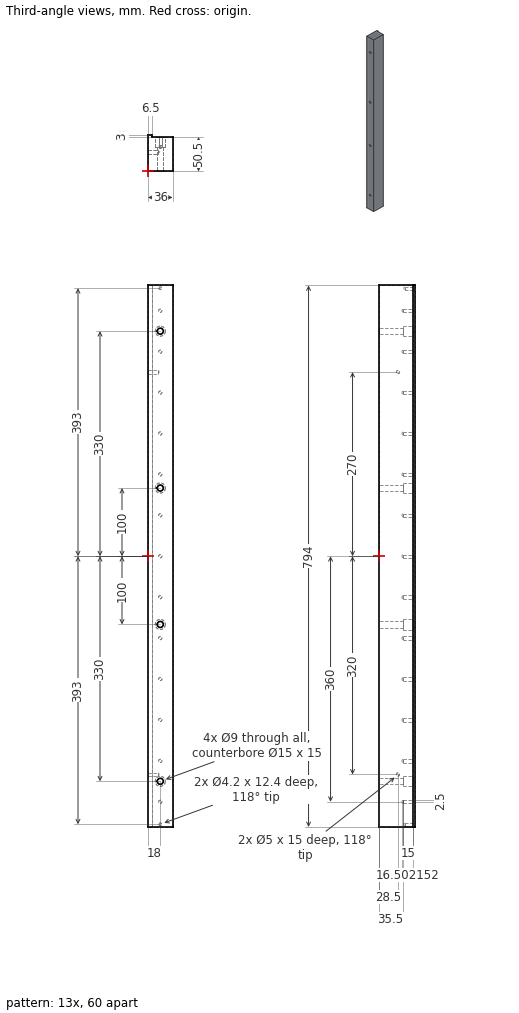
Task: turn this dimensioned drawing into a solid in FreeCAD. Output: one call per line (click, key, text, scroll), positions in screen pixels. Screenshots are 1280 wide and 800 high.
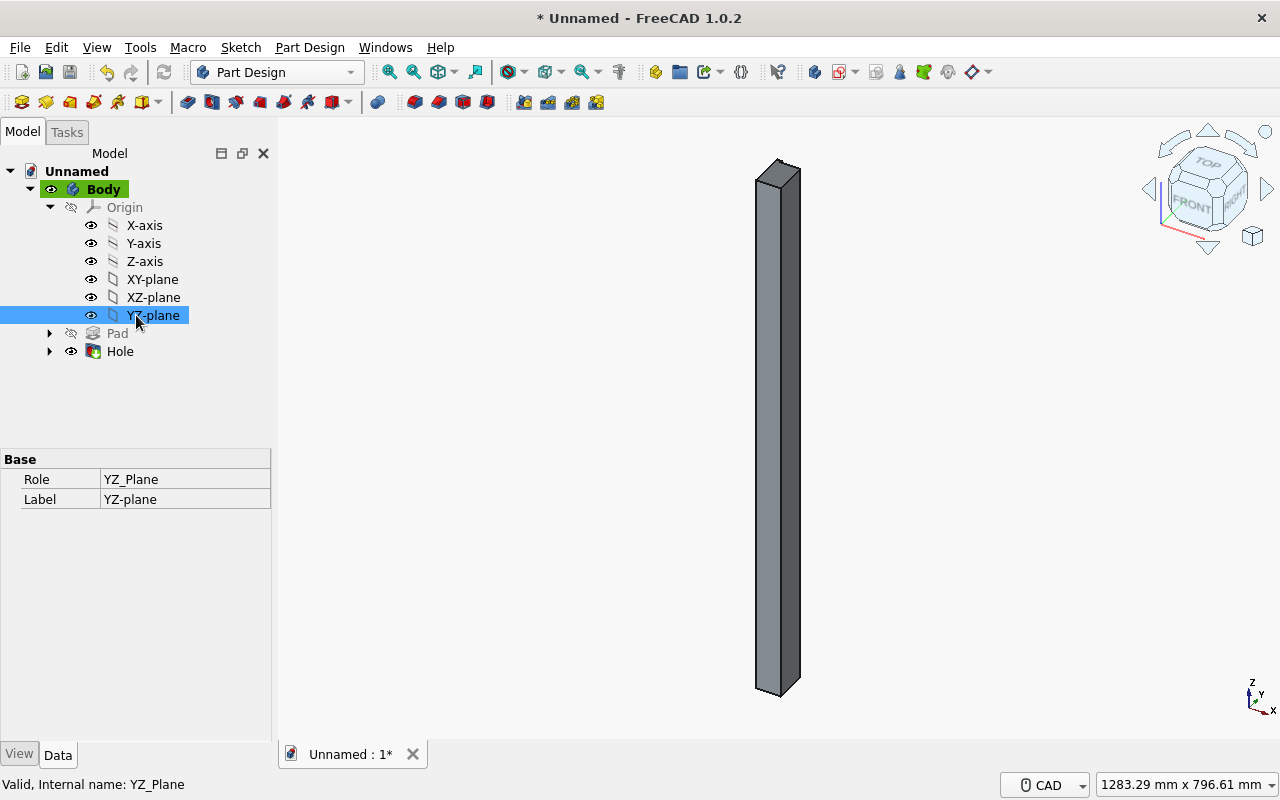
click(972, 72)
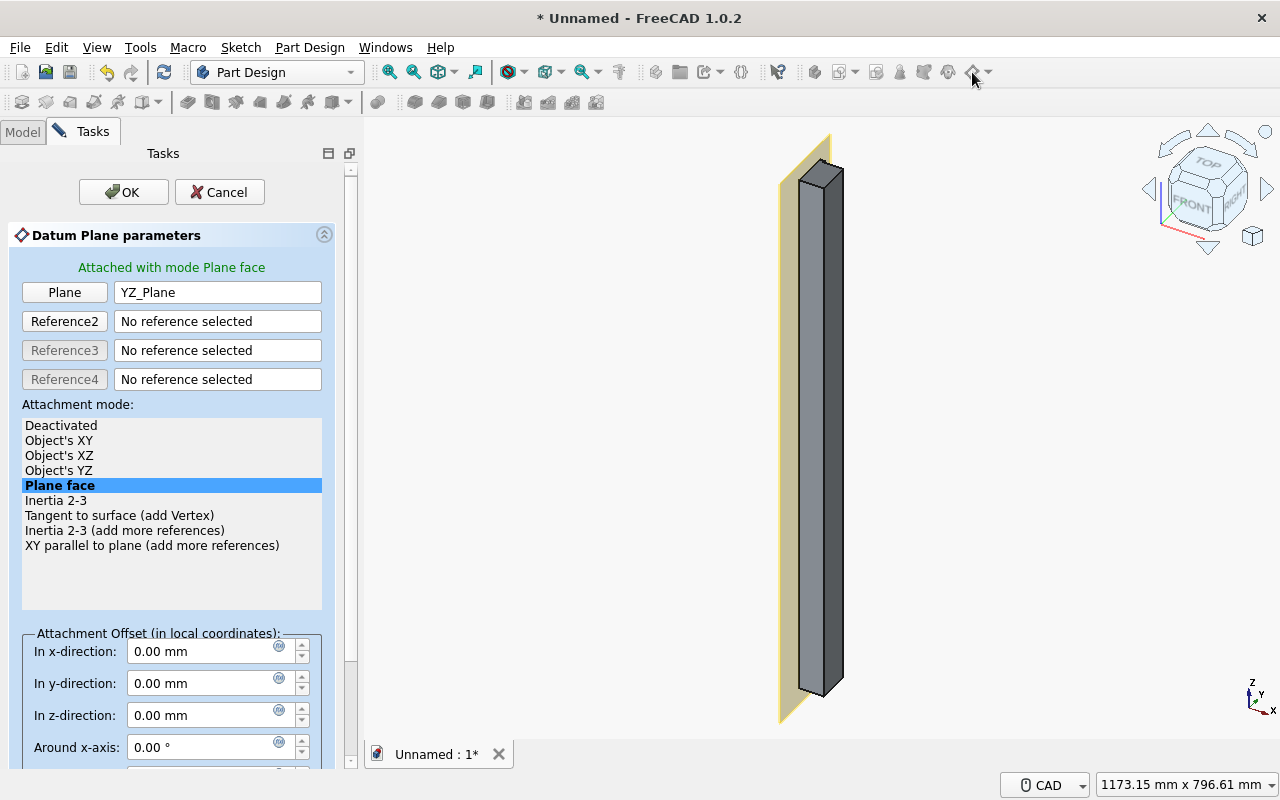
triple_click(210, 715)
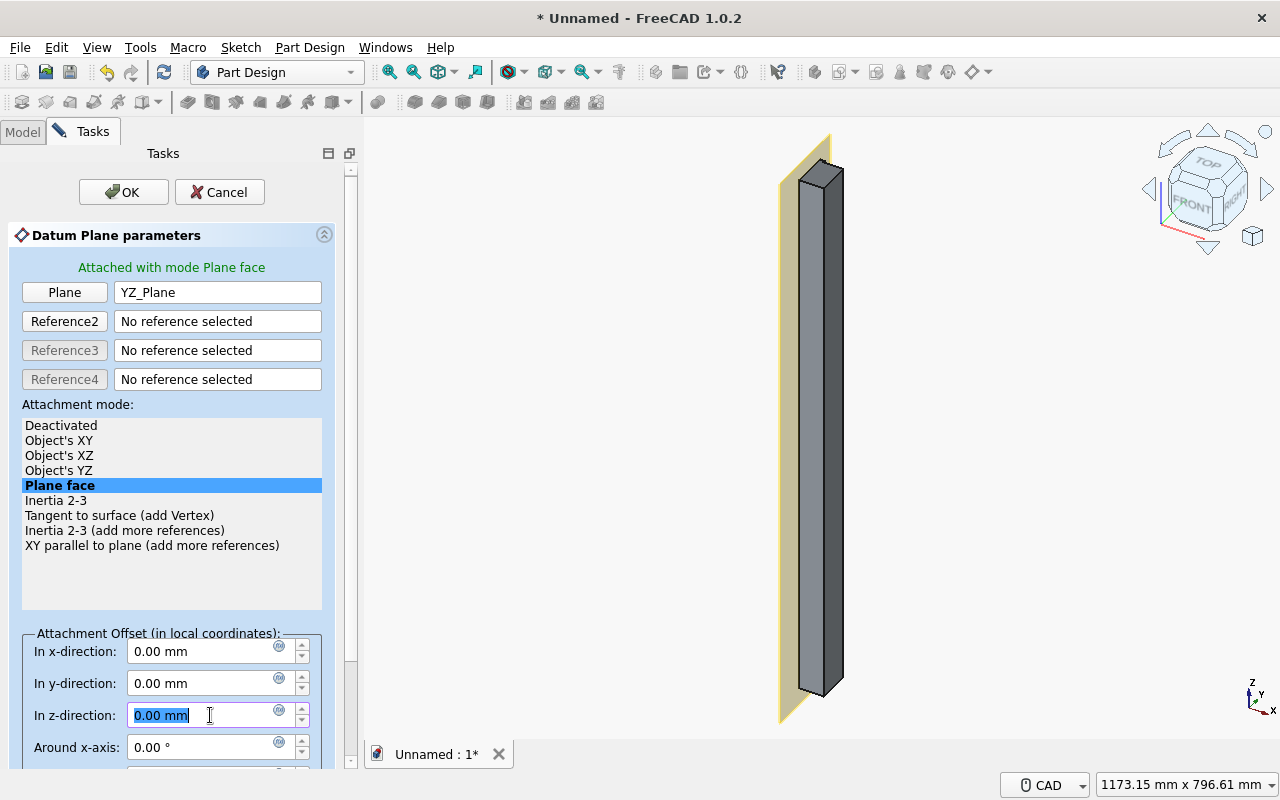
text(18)
key(Tab)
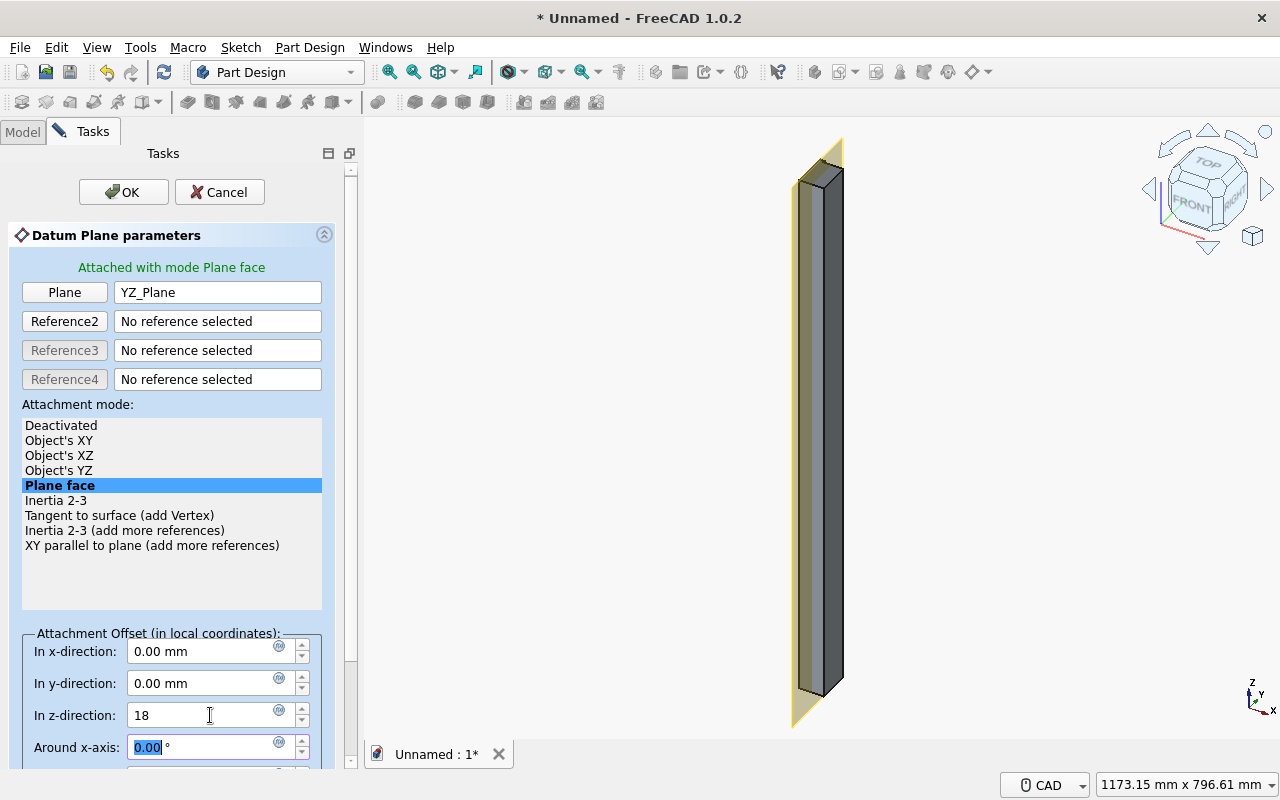
click(124, 192)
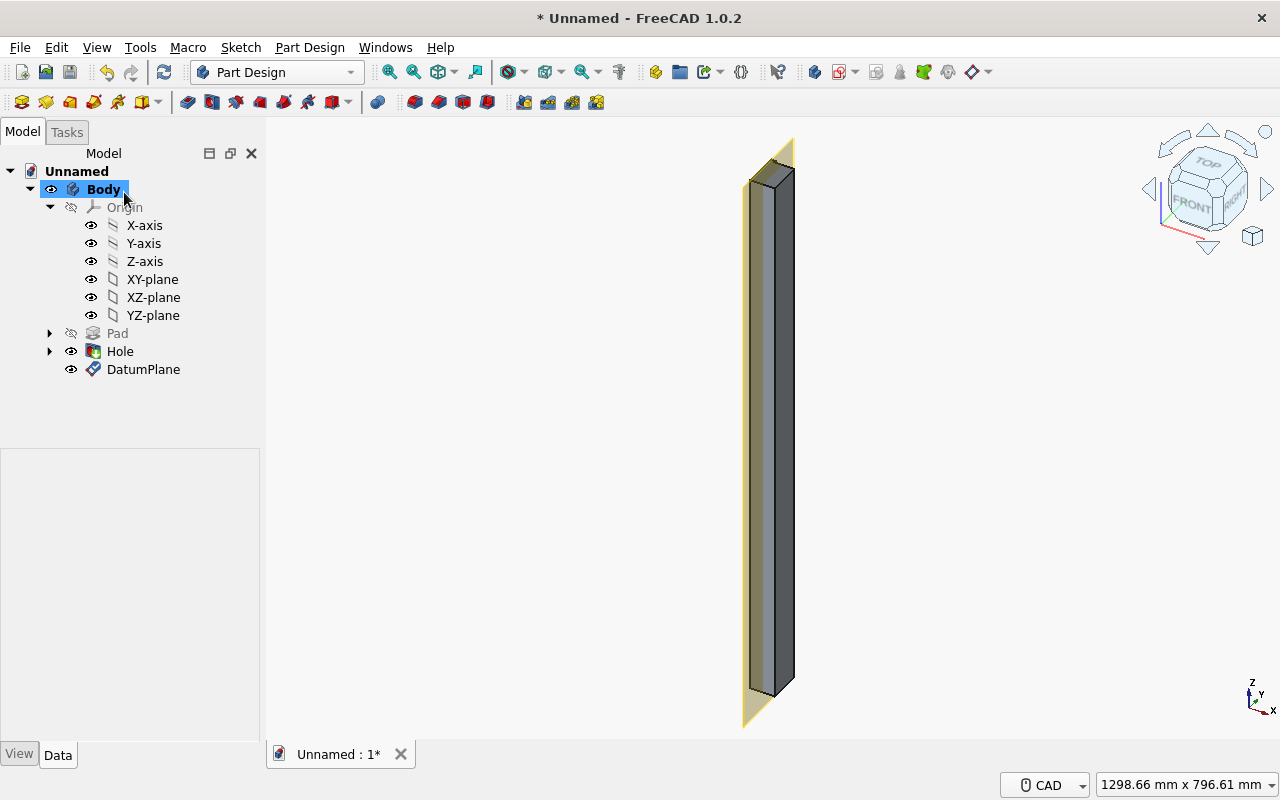
click(116, 369)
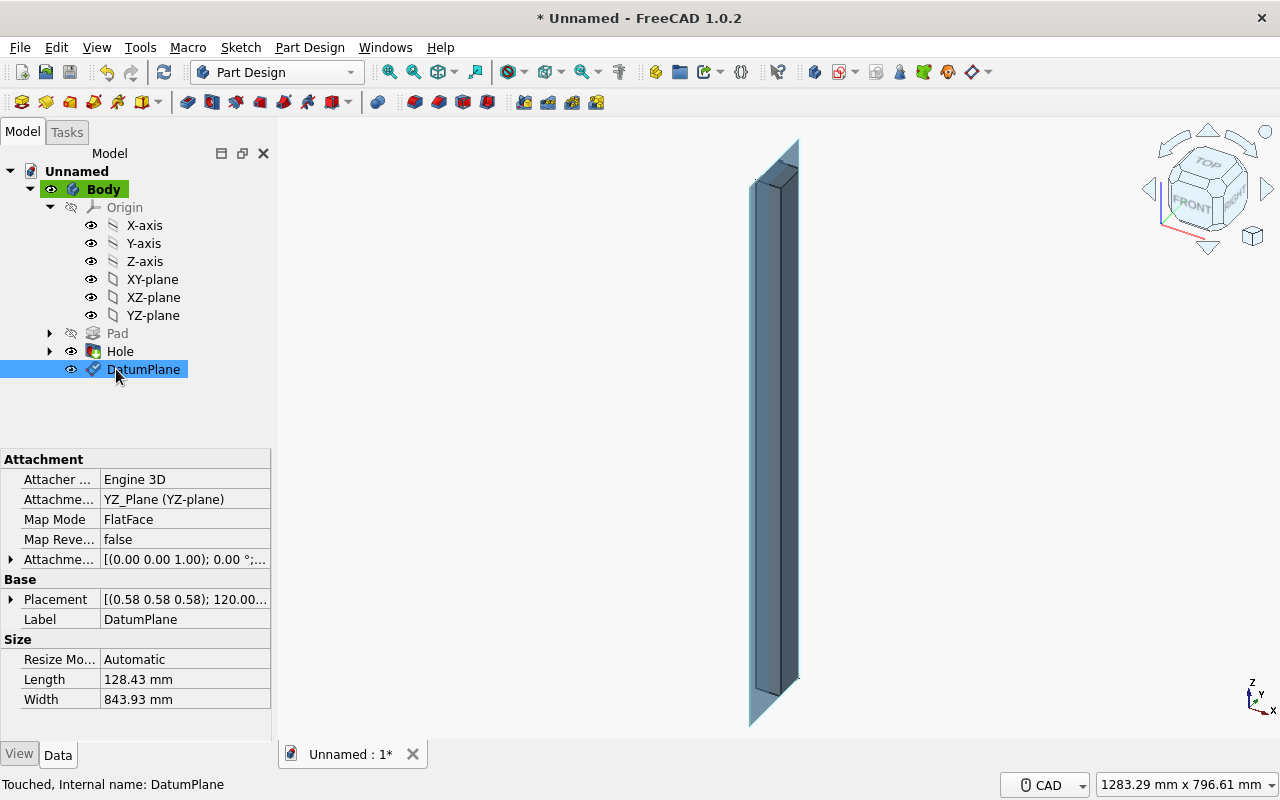
click(840, 72)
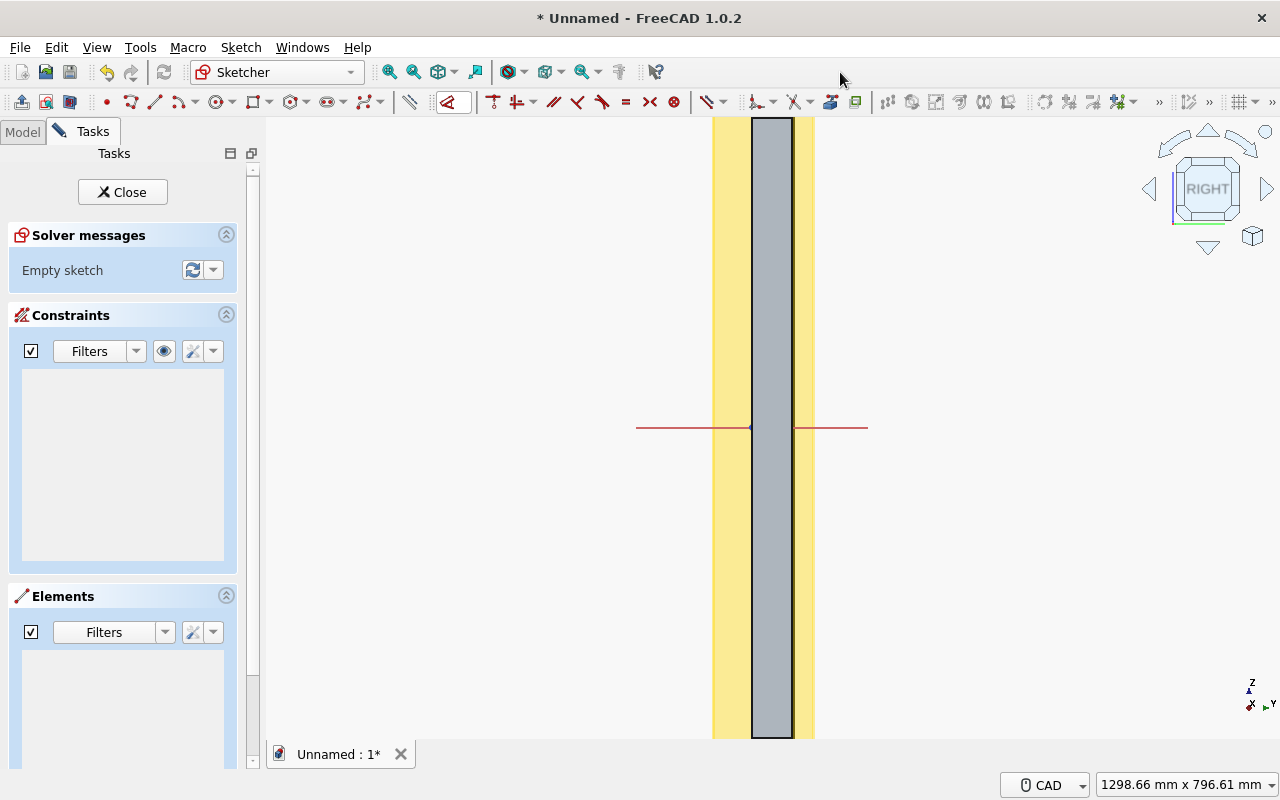
click(70, 102)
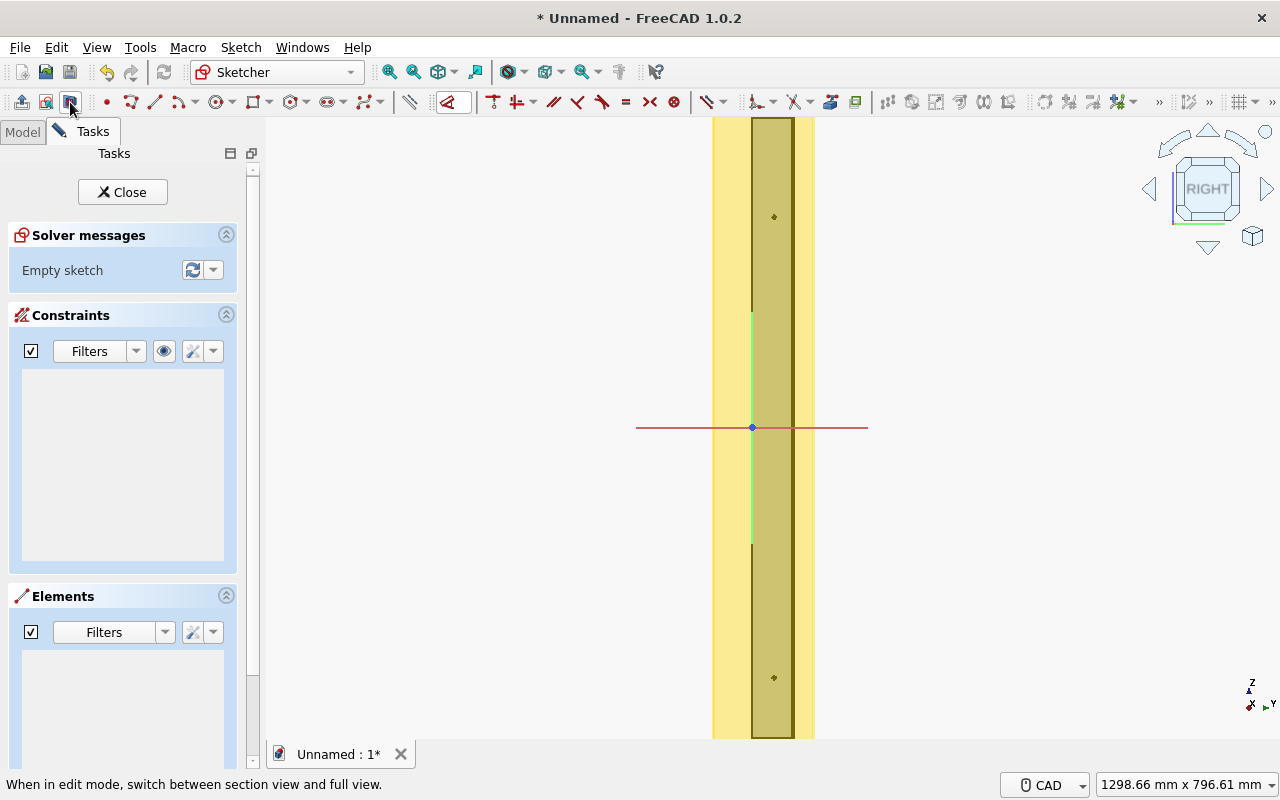
scroll(787, 711, up, 15)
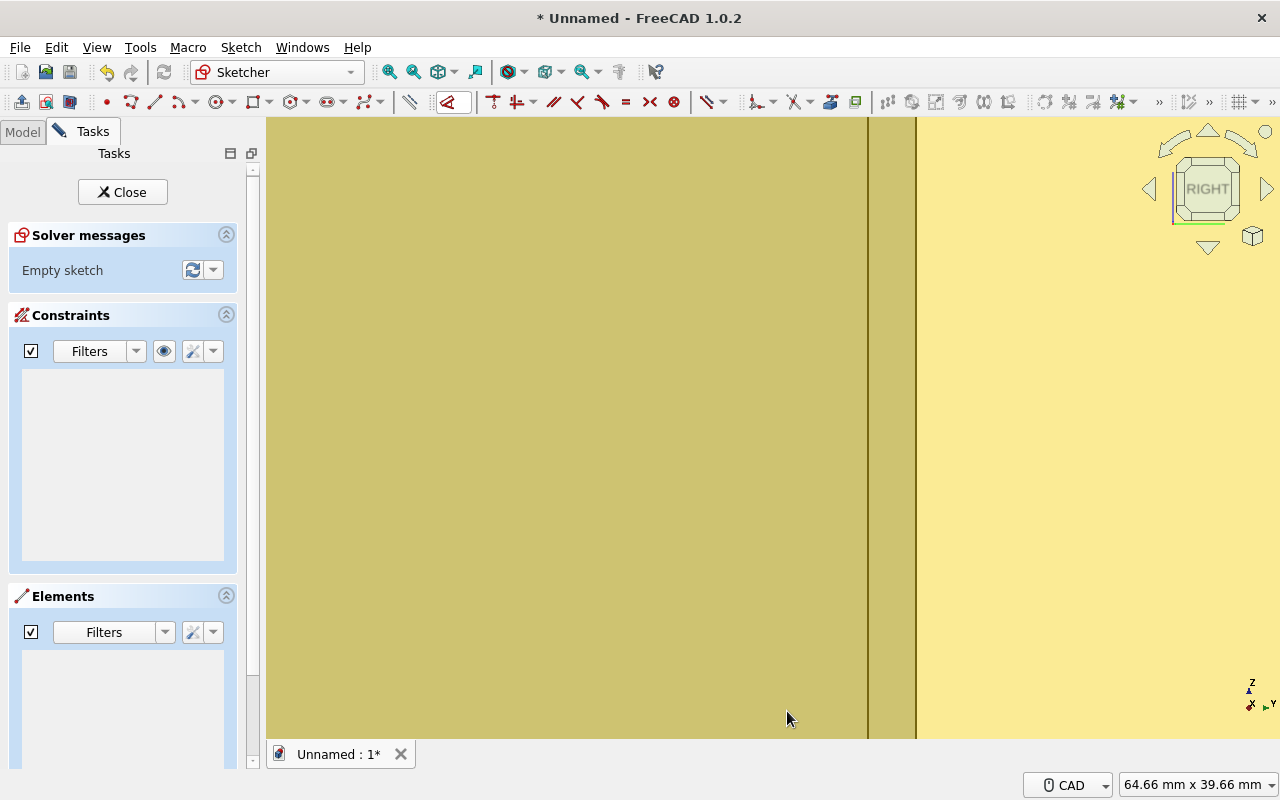
scroll(652, 711, up, 2)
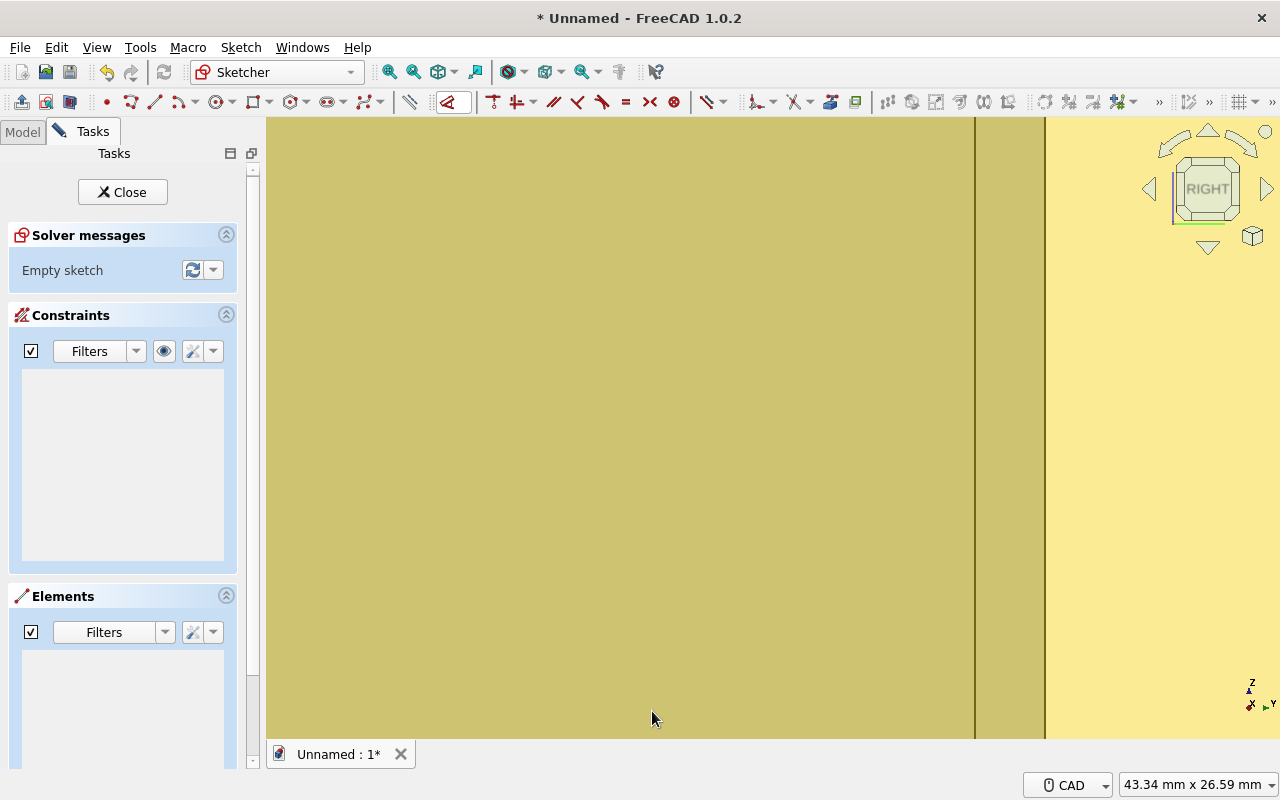
click(132, 102)